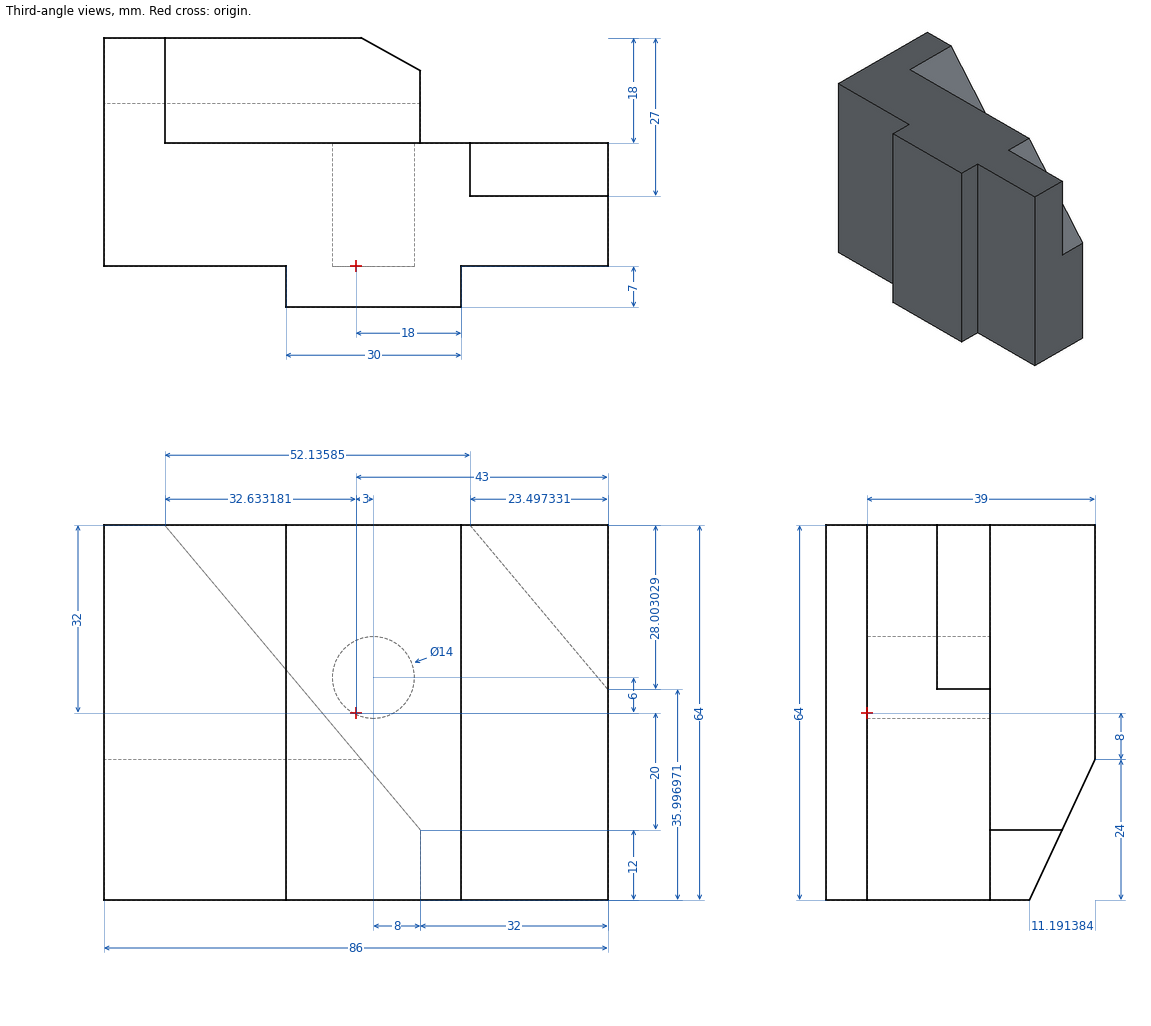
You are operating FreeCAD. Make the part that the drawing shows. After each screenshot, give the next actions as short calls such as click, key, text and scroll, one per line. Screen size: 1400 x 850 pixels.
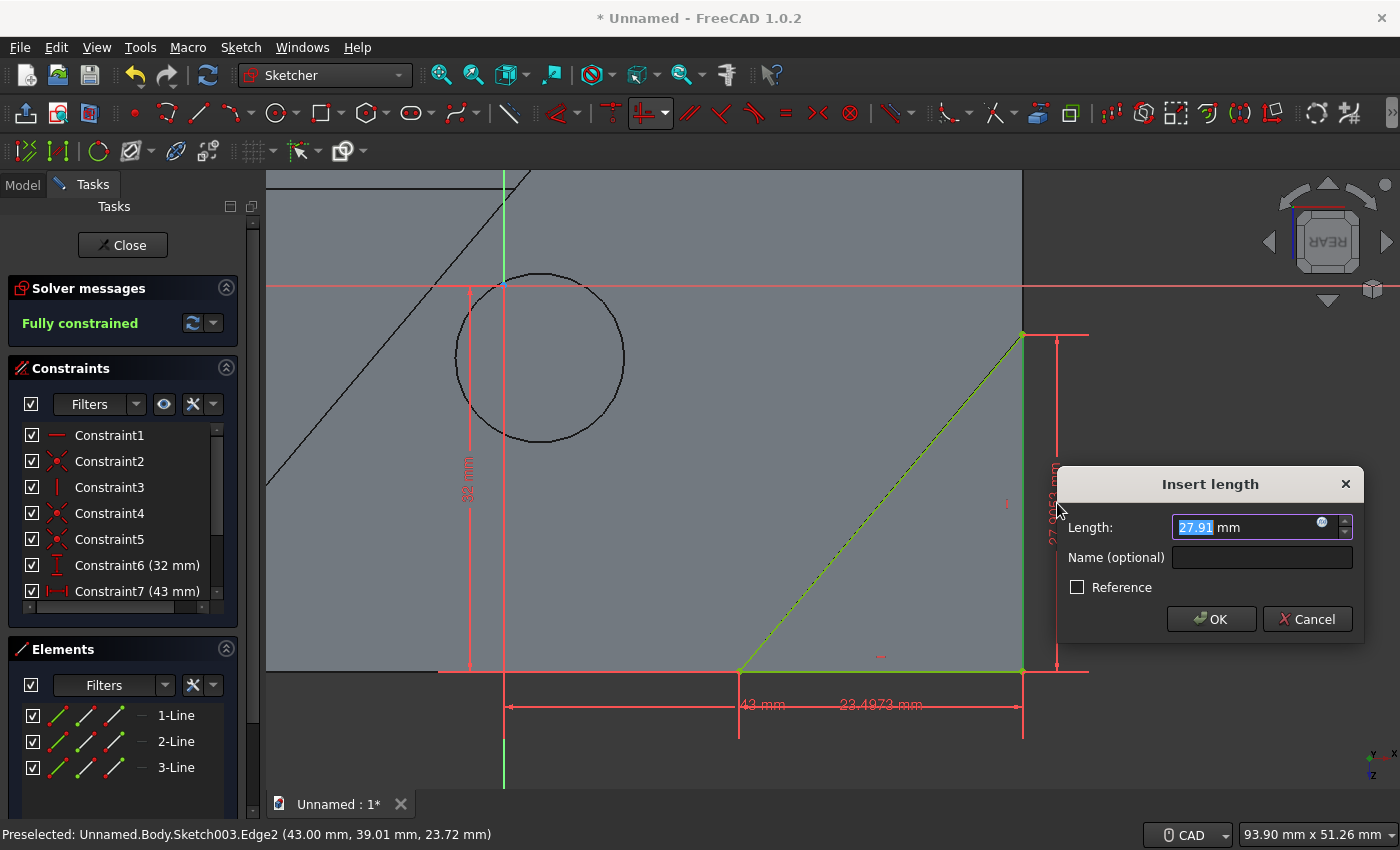
text(28.003029)
key(Return)
key(Escape)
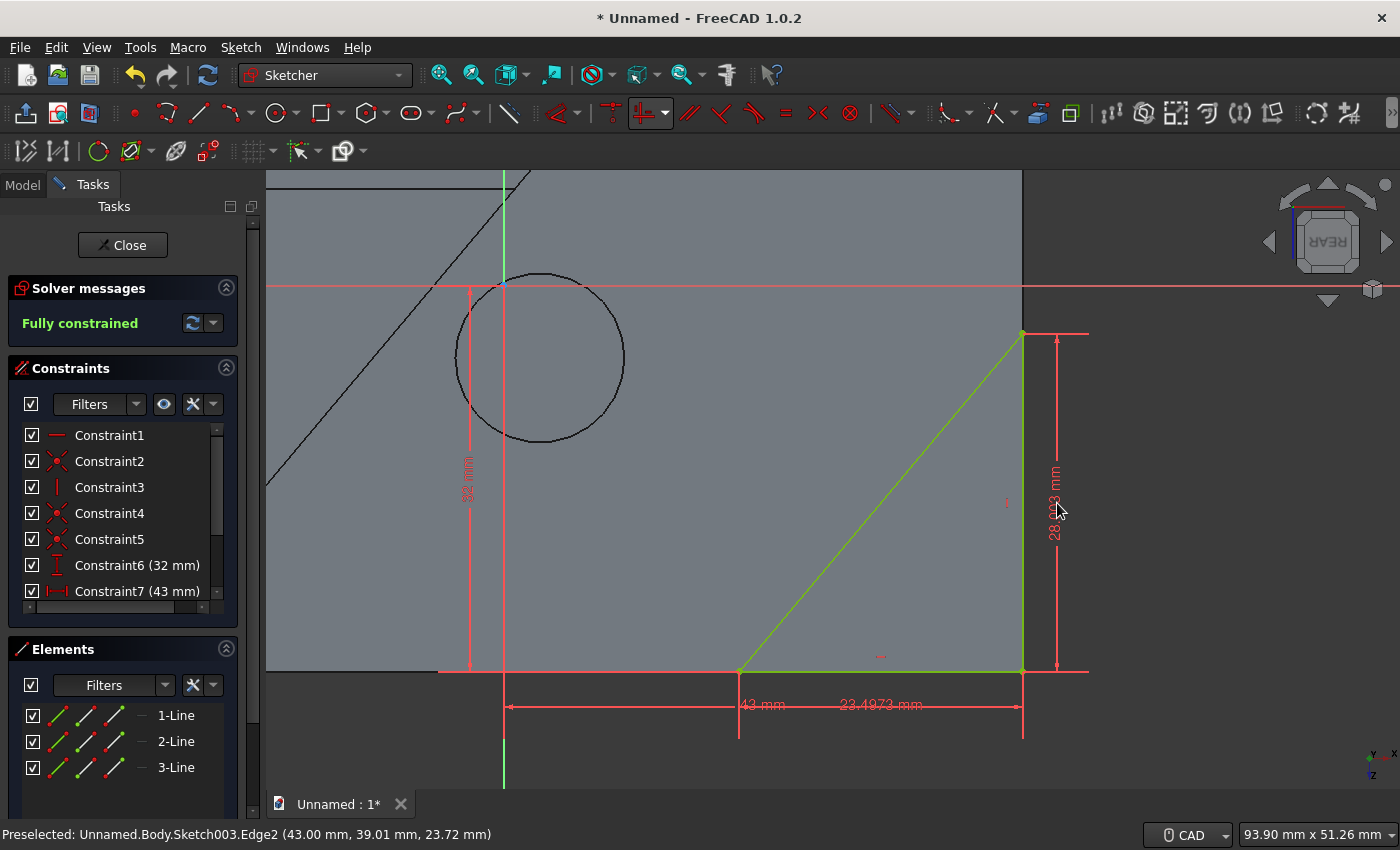
click(123, 245)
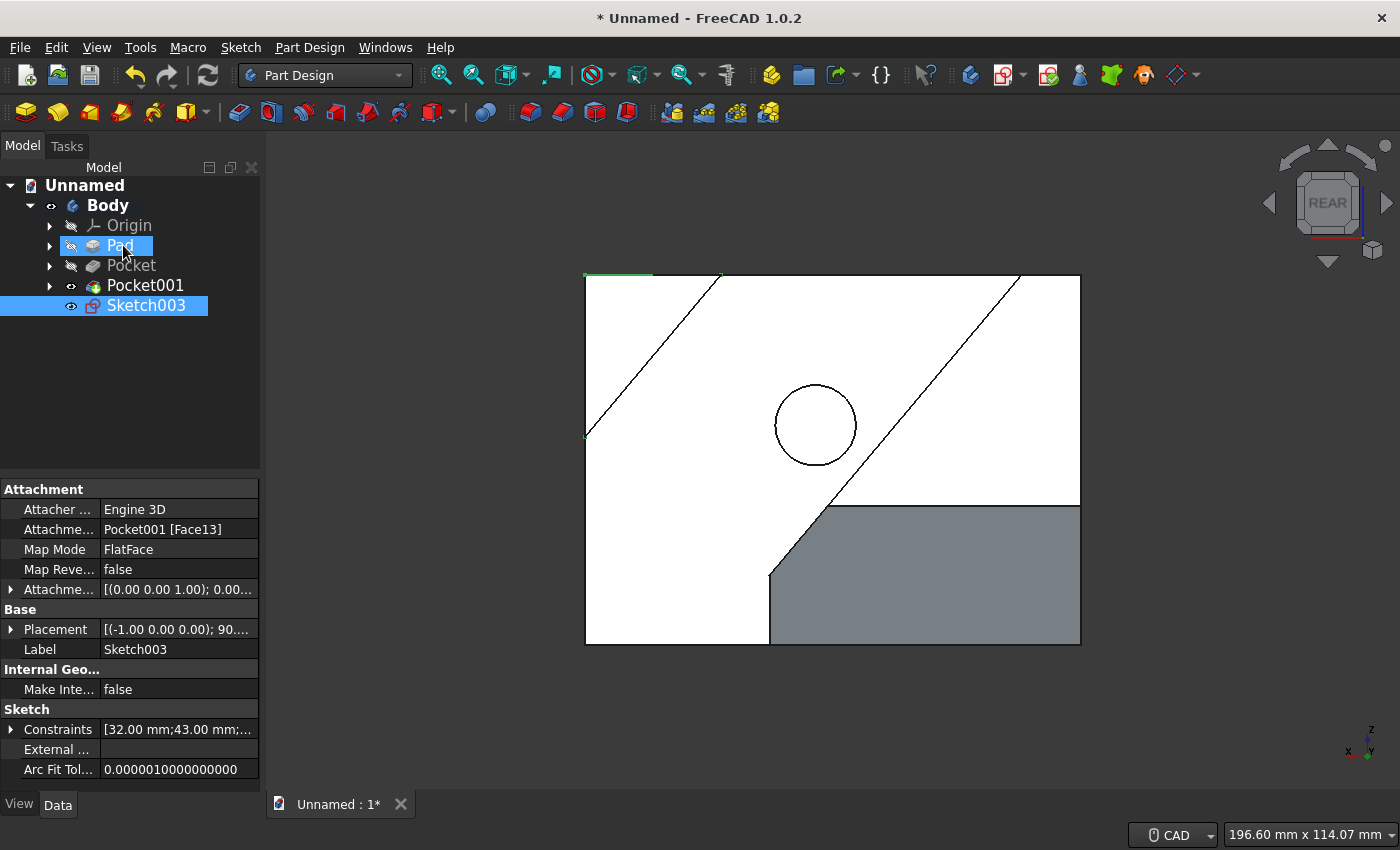
click(240, 112)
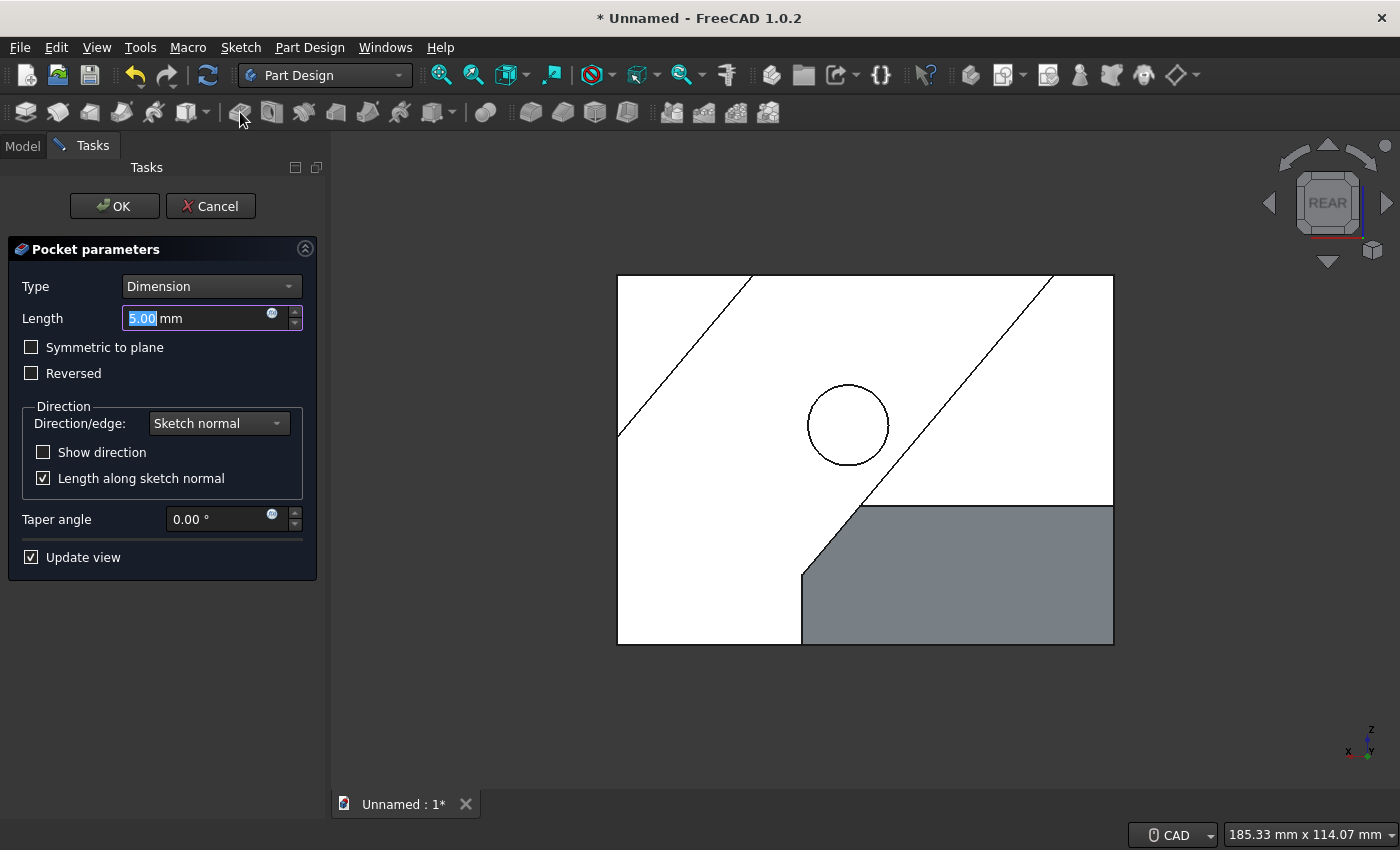
text(27)
key(Tab)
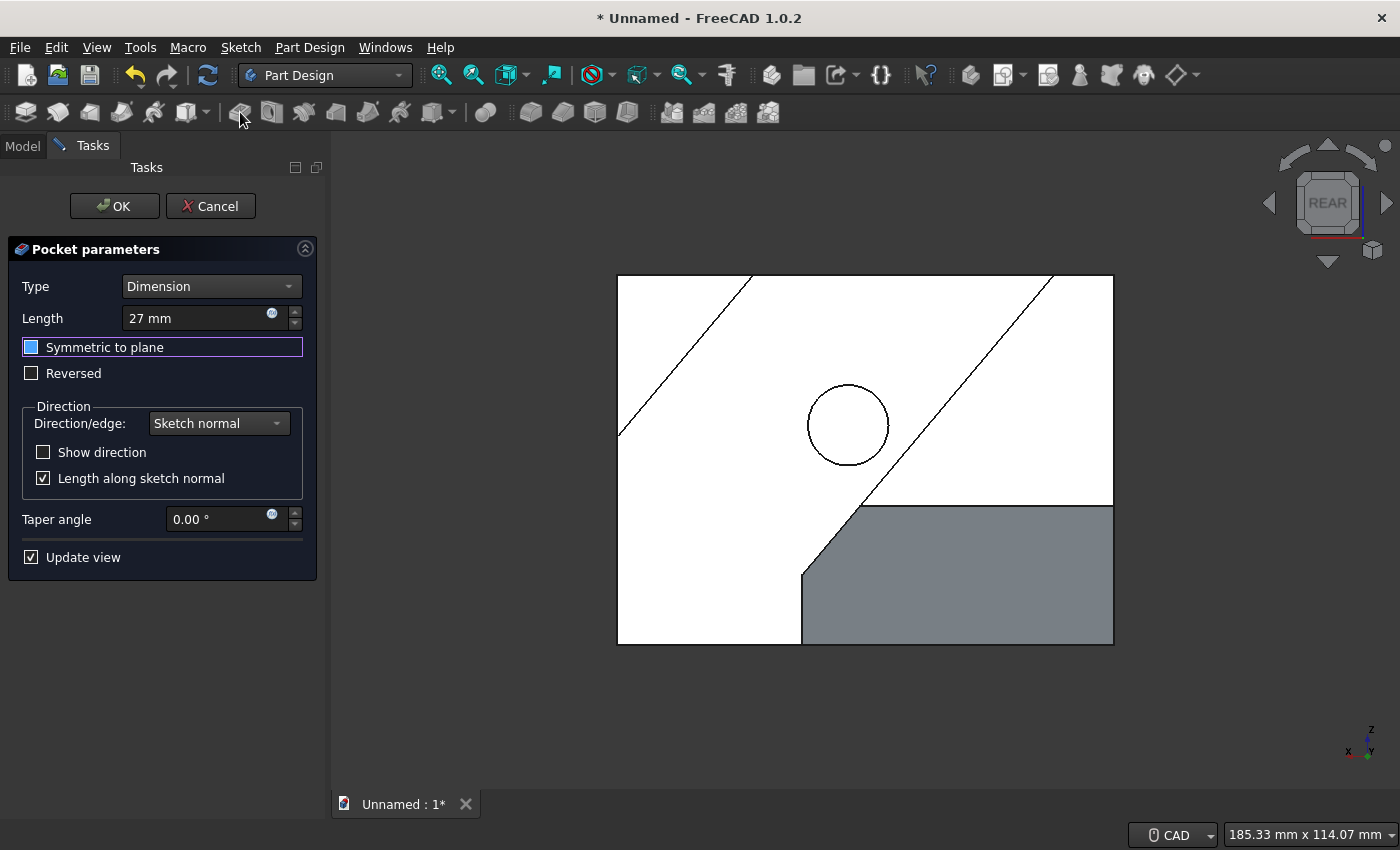
click(115, 206)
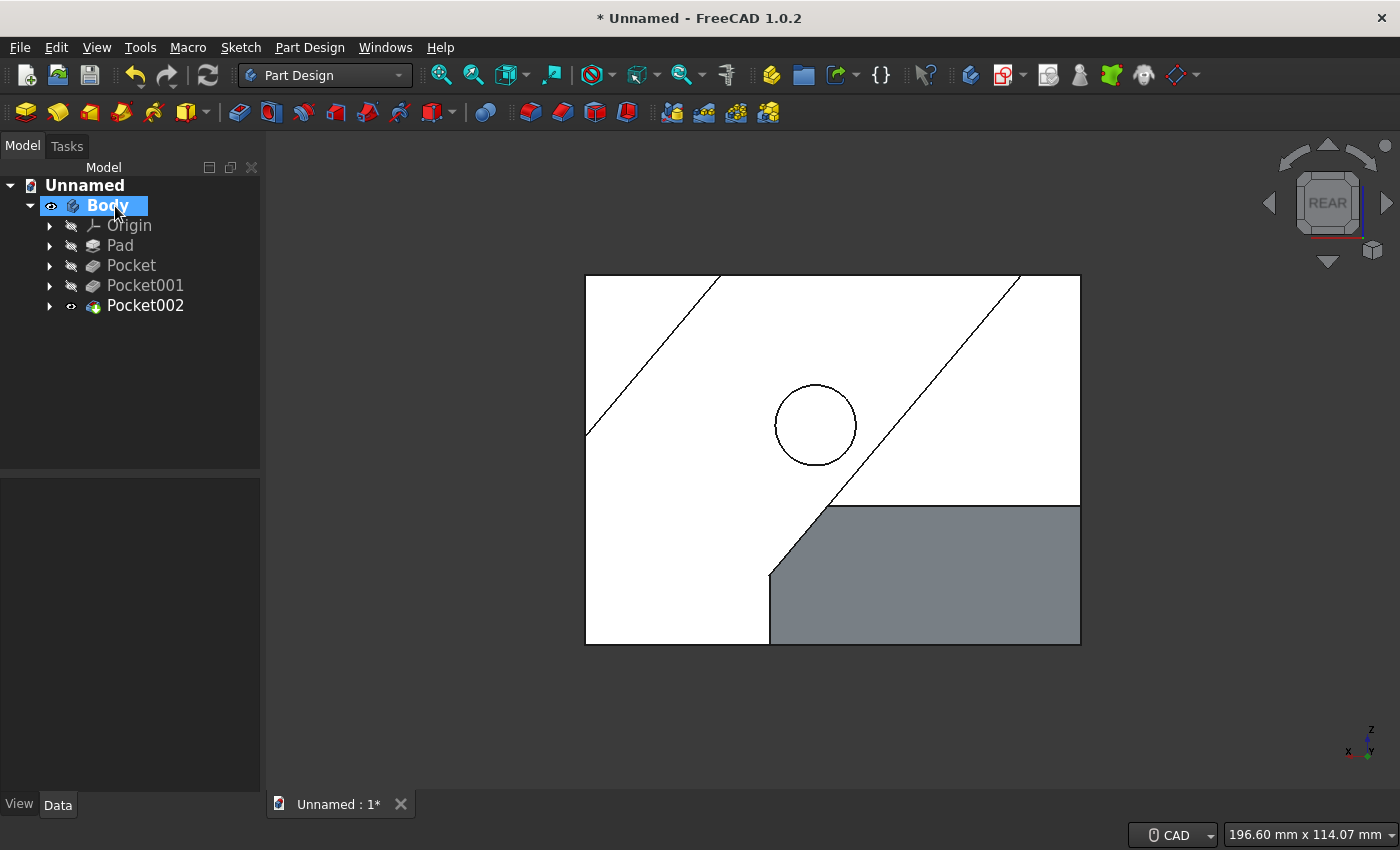
click(991, 423)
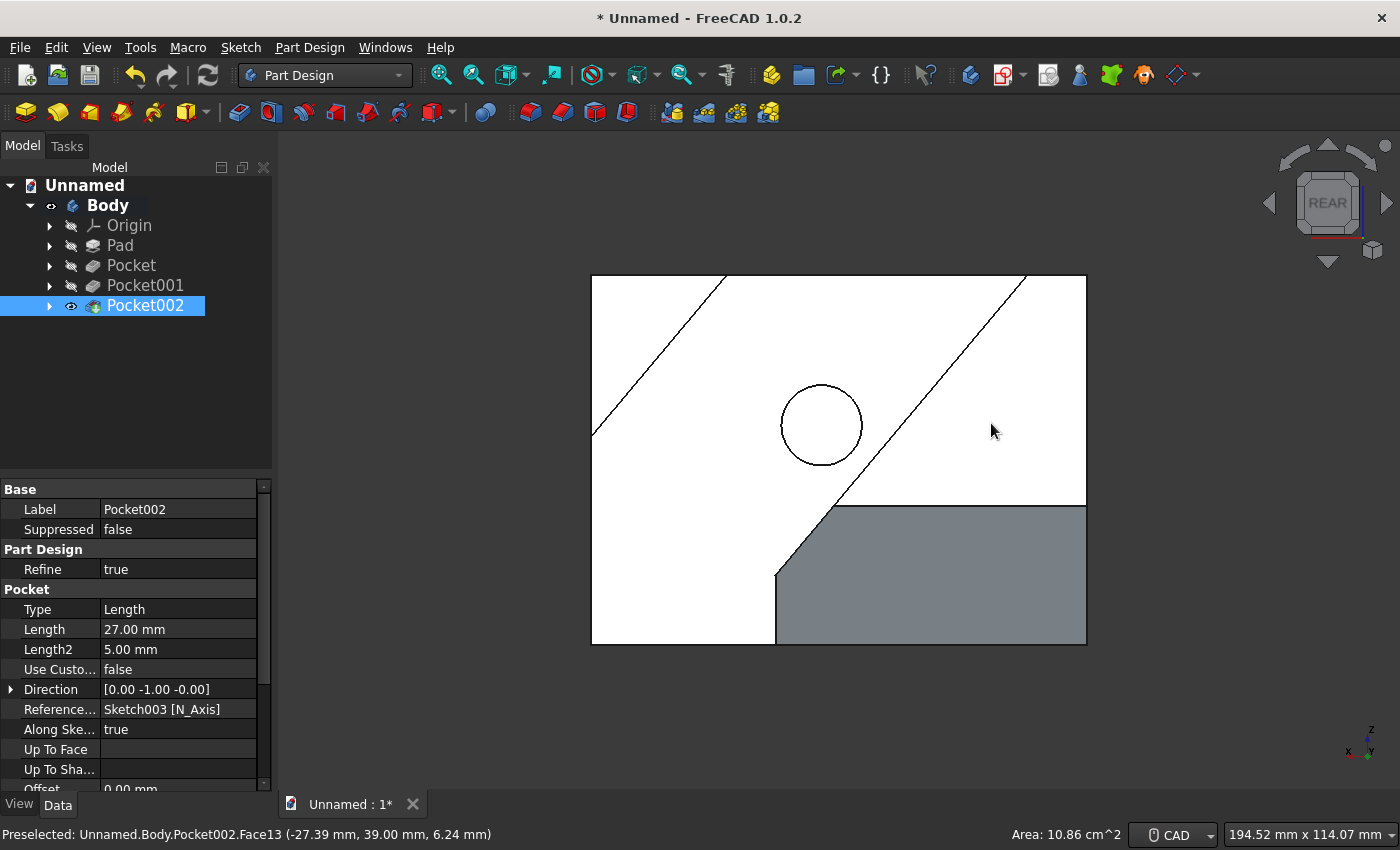
click(1004, 76)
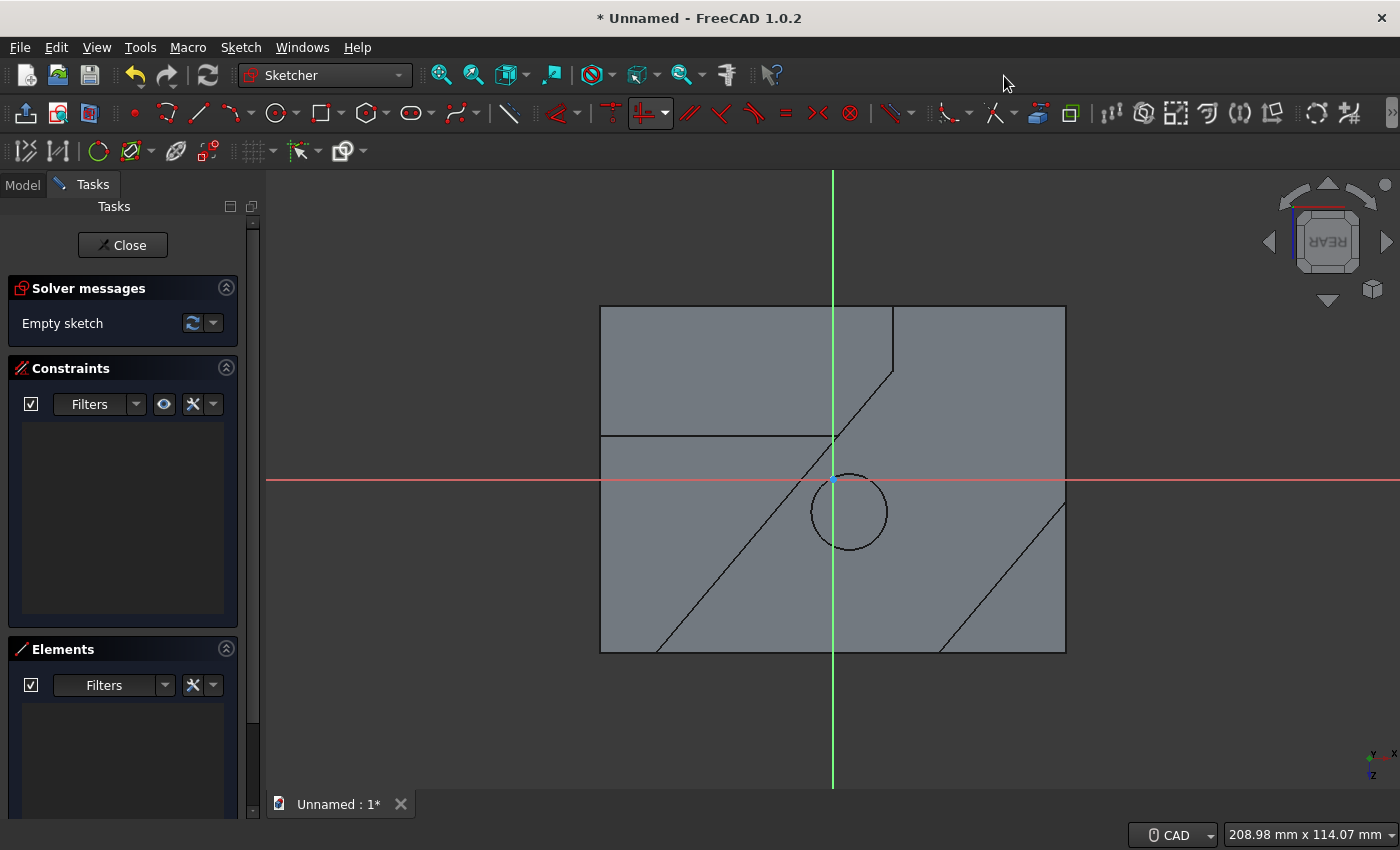
scroll(871, 520, up, 8)